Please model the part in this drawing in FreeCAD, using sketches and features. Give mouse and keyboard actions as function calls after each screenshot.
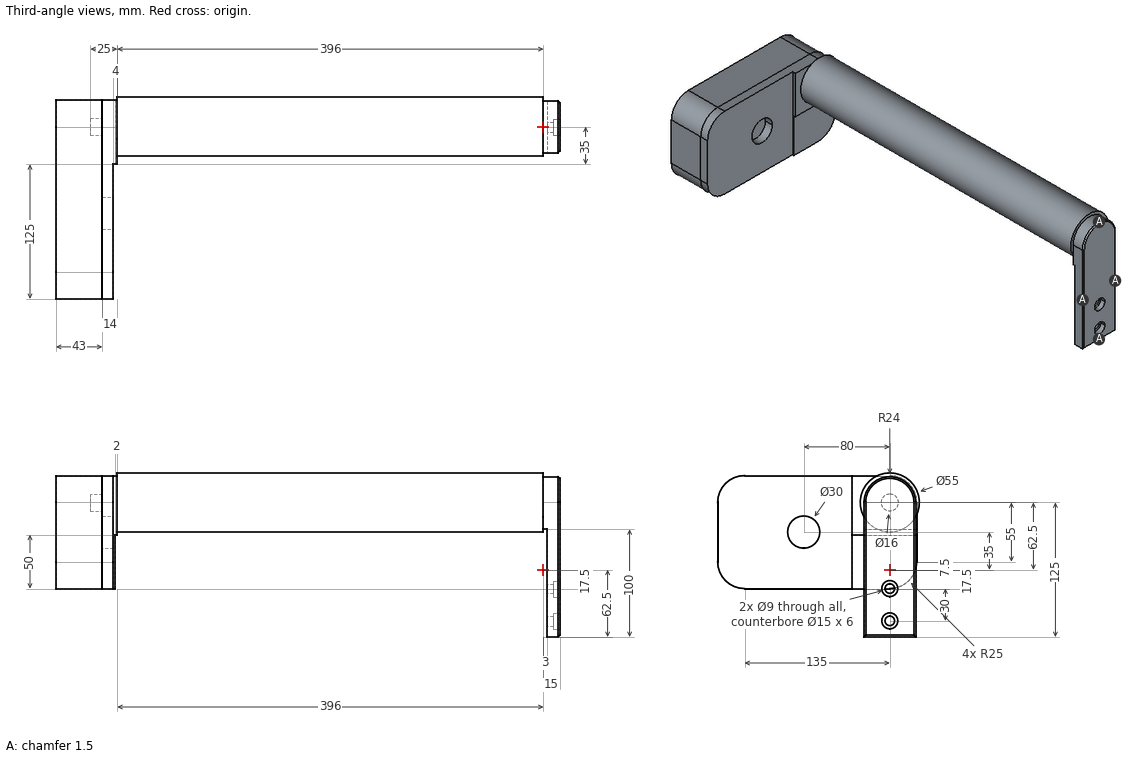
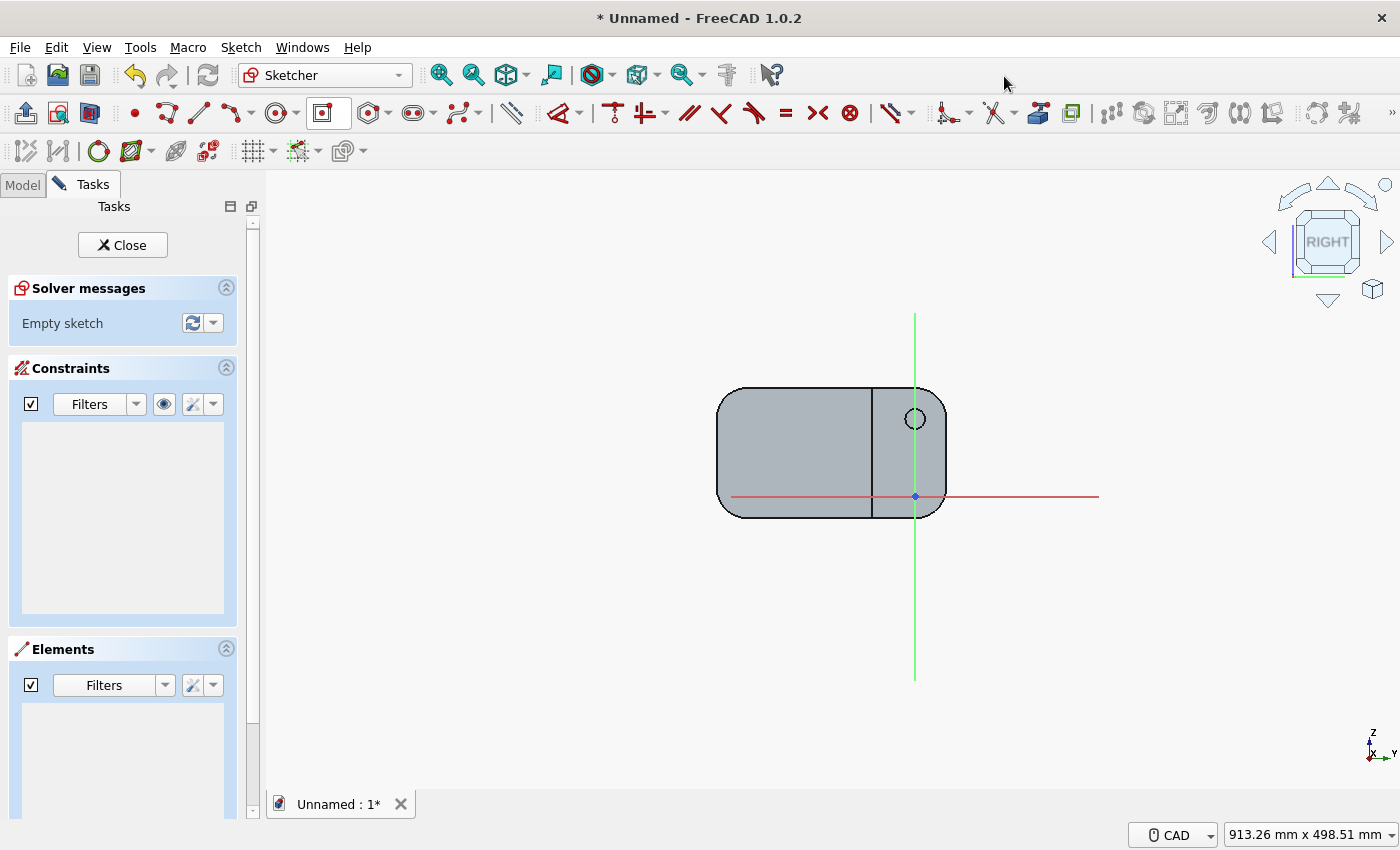
scroll(821, 450, up, 12)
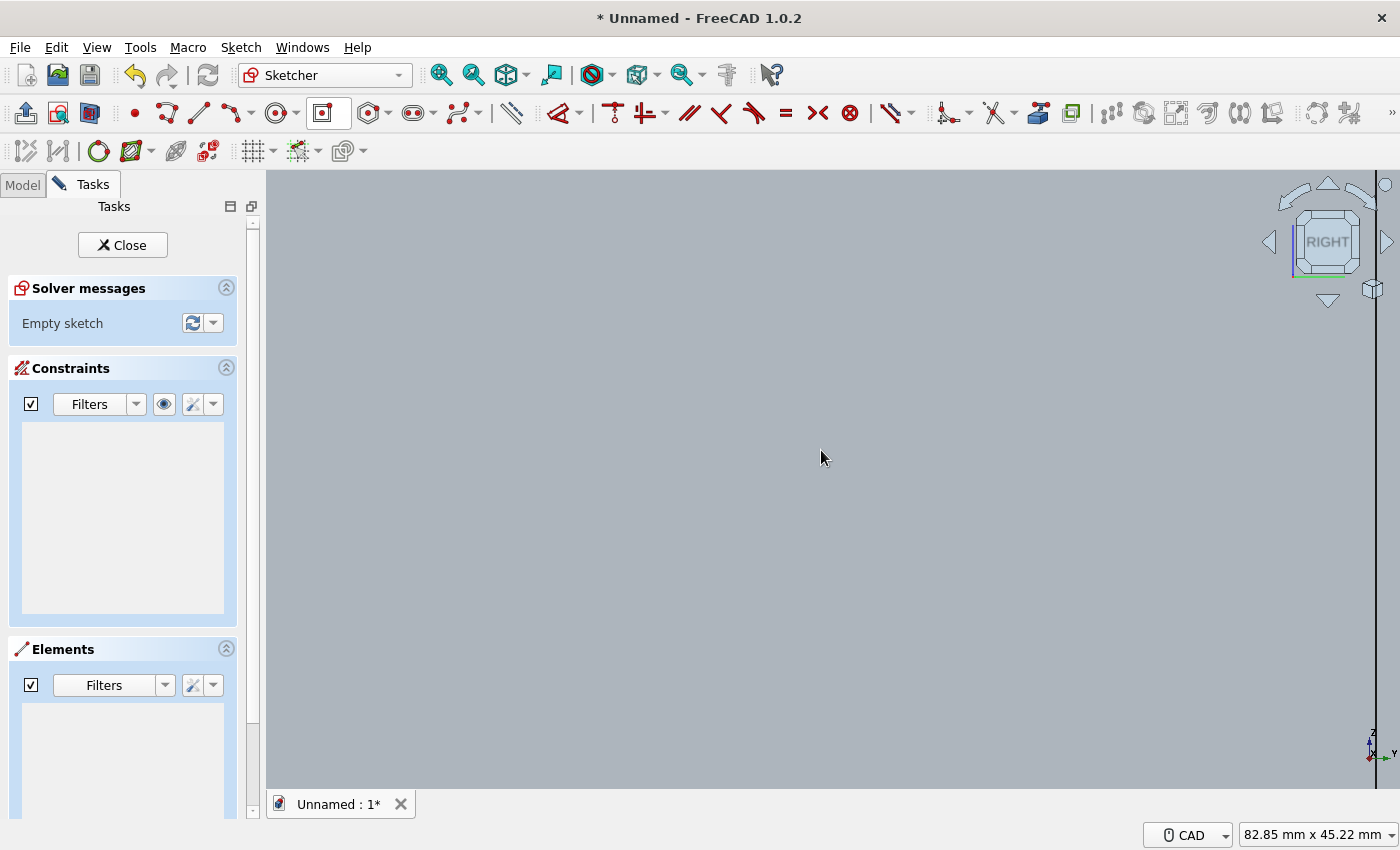
key(g)
key(c)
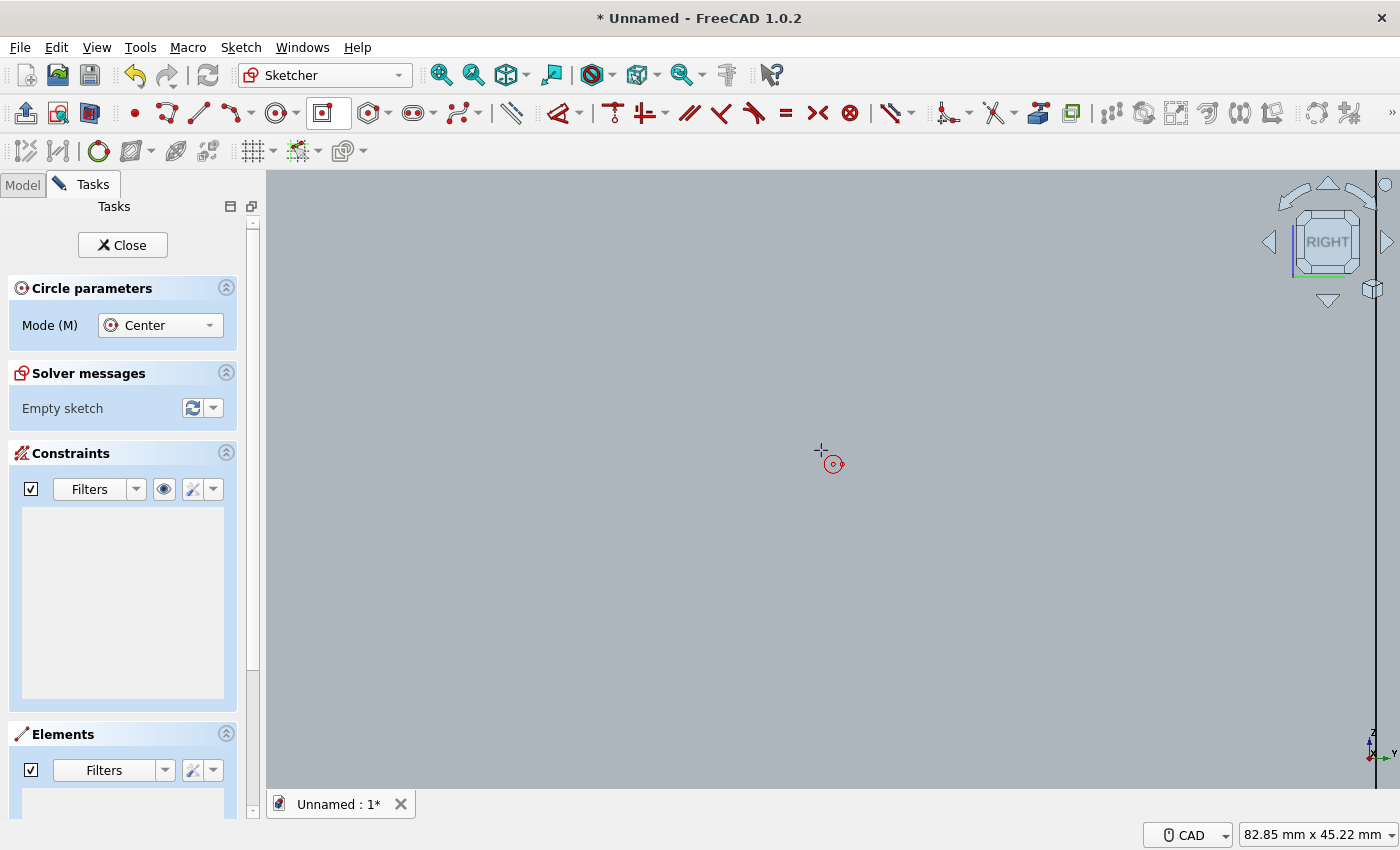
click(760, 480)
move(905, 335)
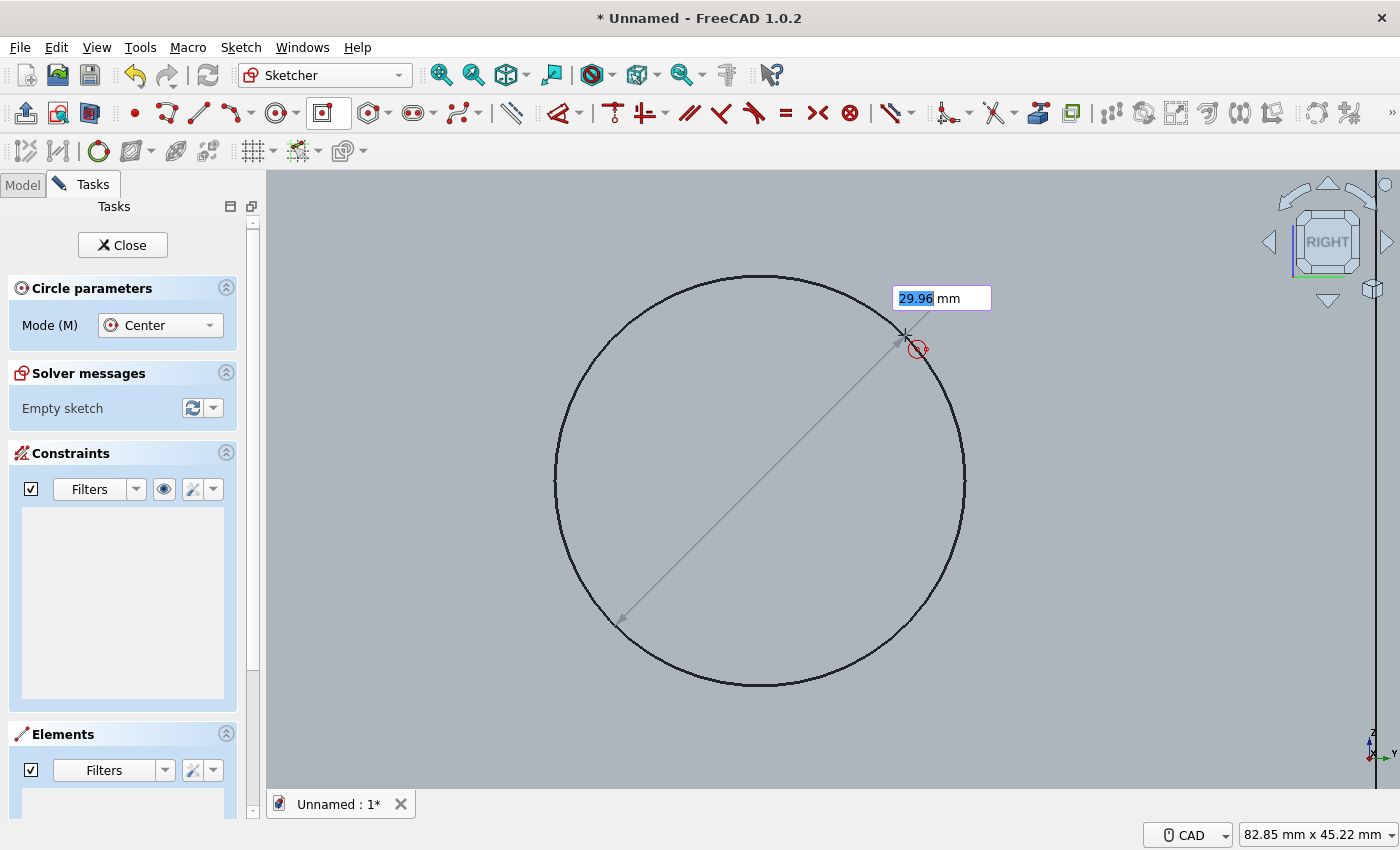
text(30)
key(Return)
key(Escape)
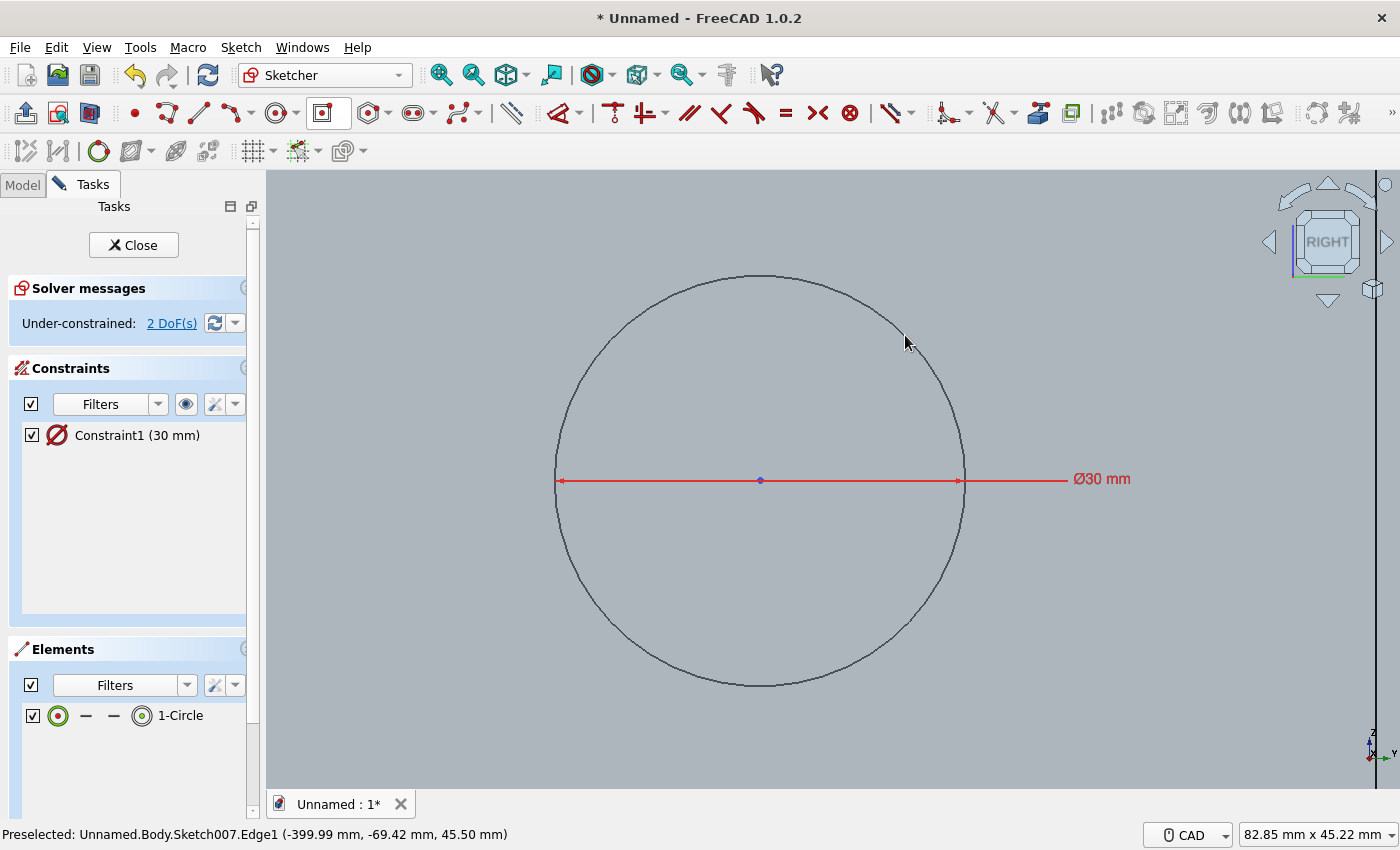
key(d)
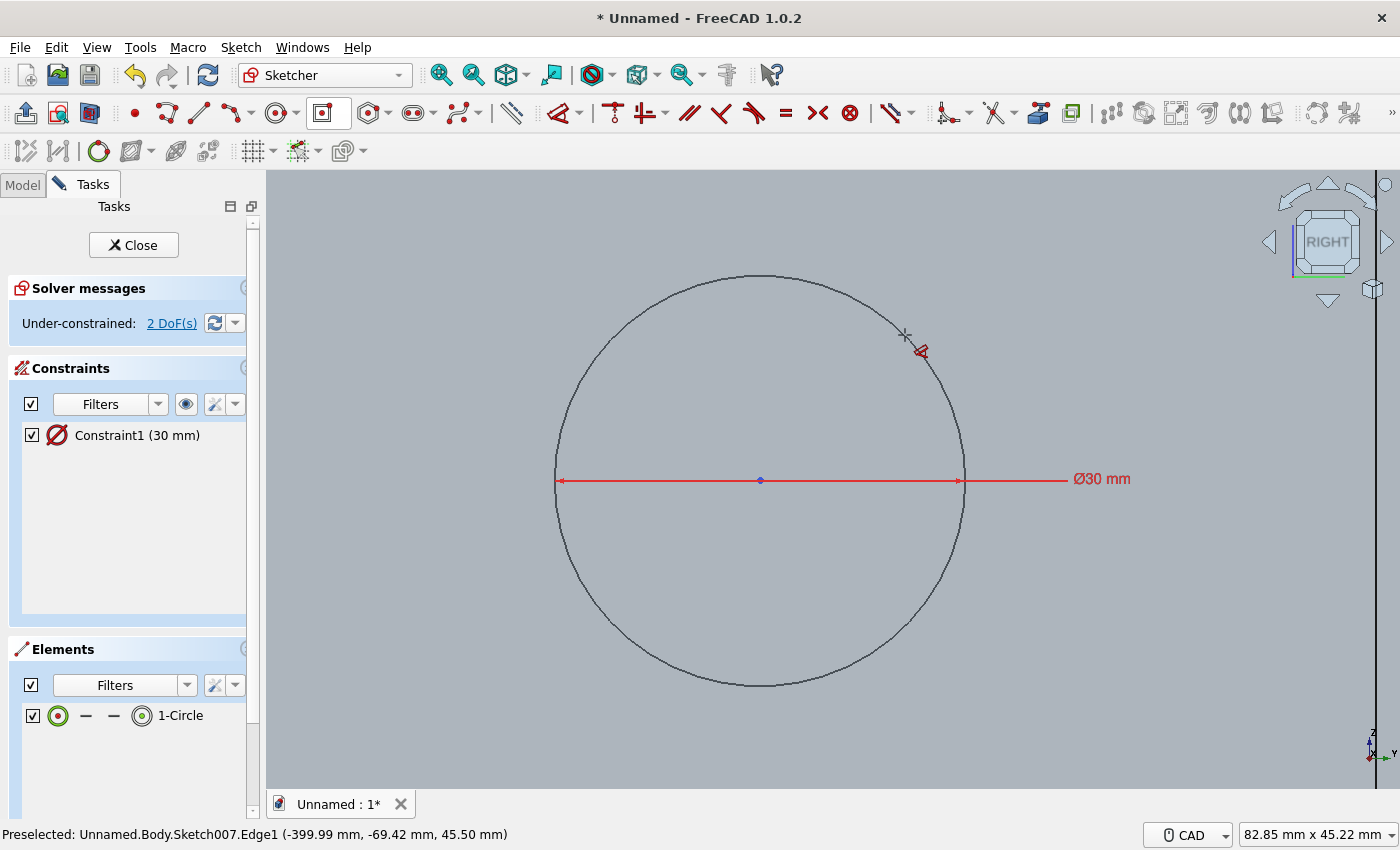
click(760, 481)
click(998, 447)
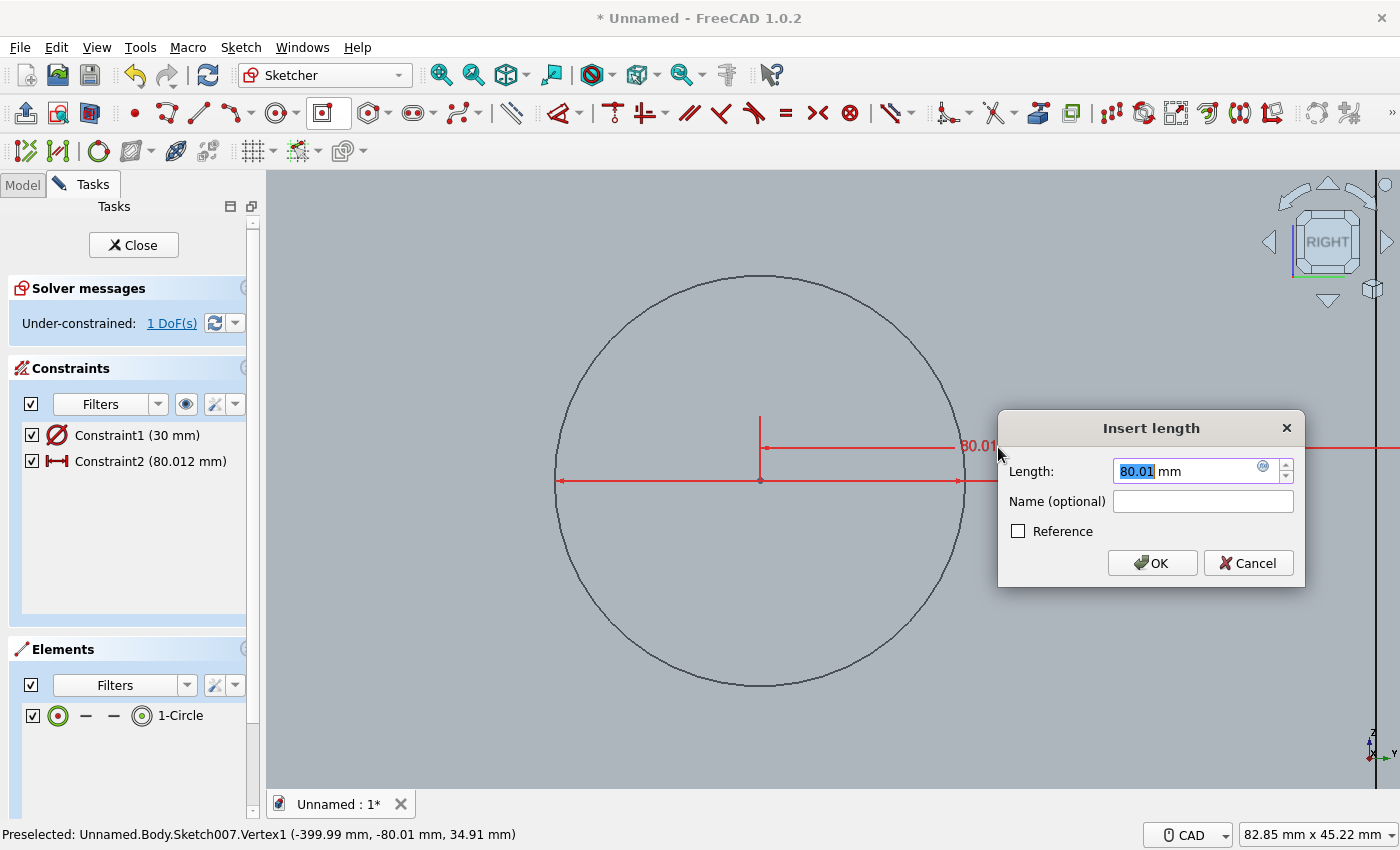
text(80)
key(Return)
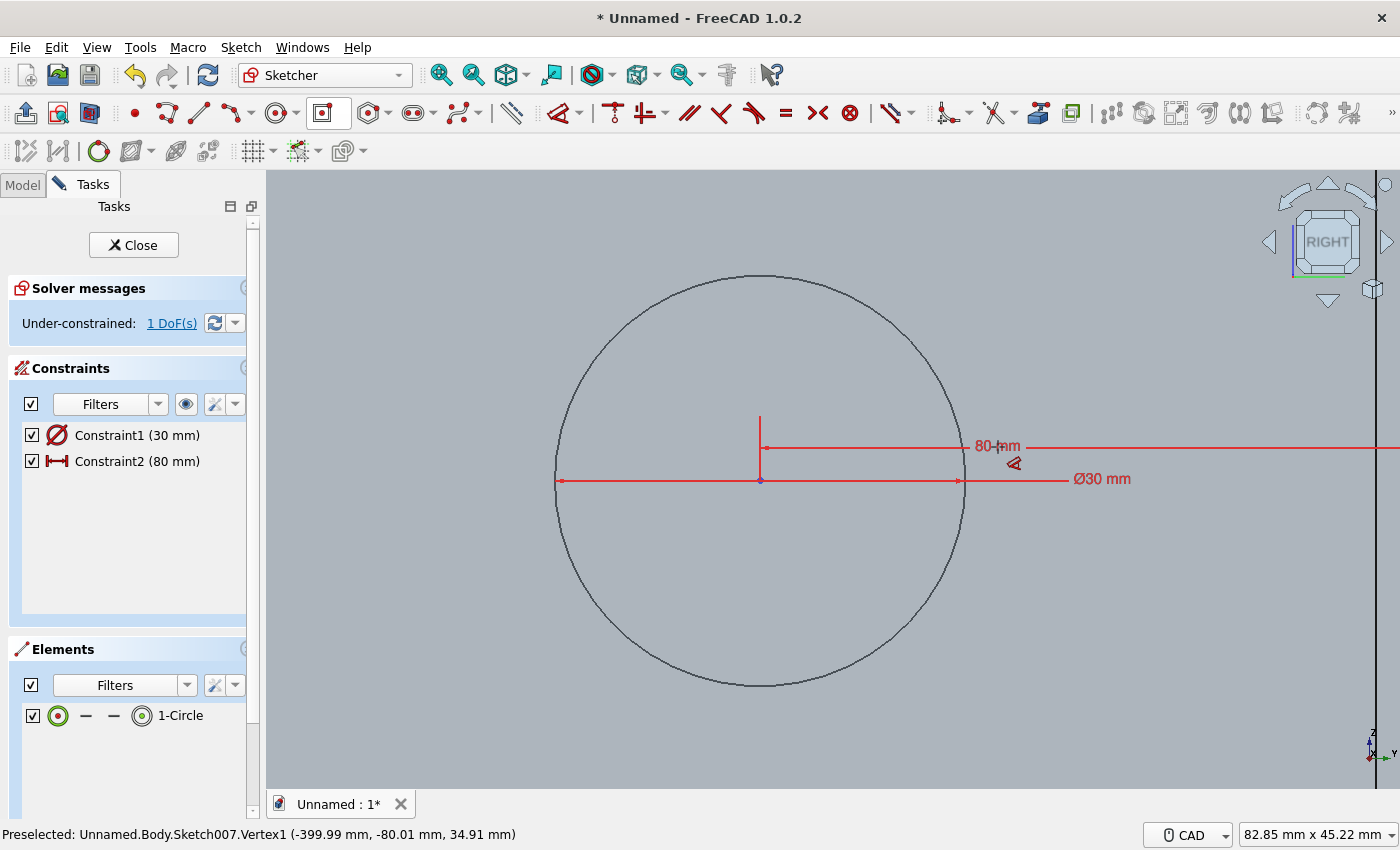
click(760, 481)
click(726, 621)